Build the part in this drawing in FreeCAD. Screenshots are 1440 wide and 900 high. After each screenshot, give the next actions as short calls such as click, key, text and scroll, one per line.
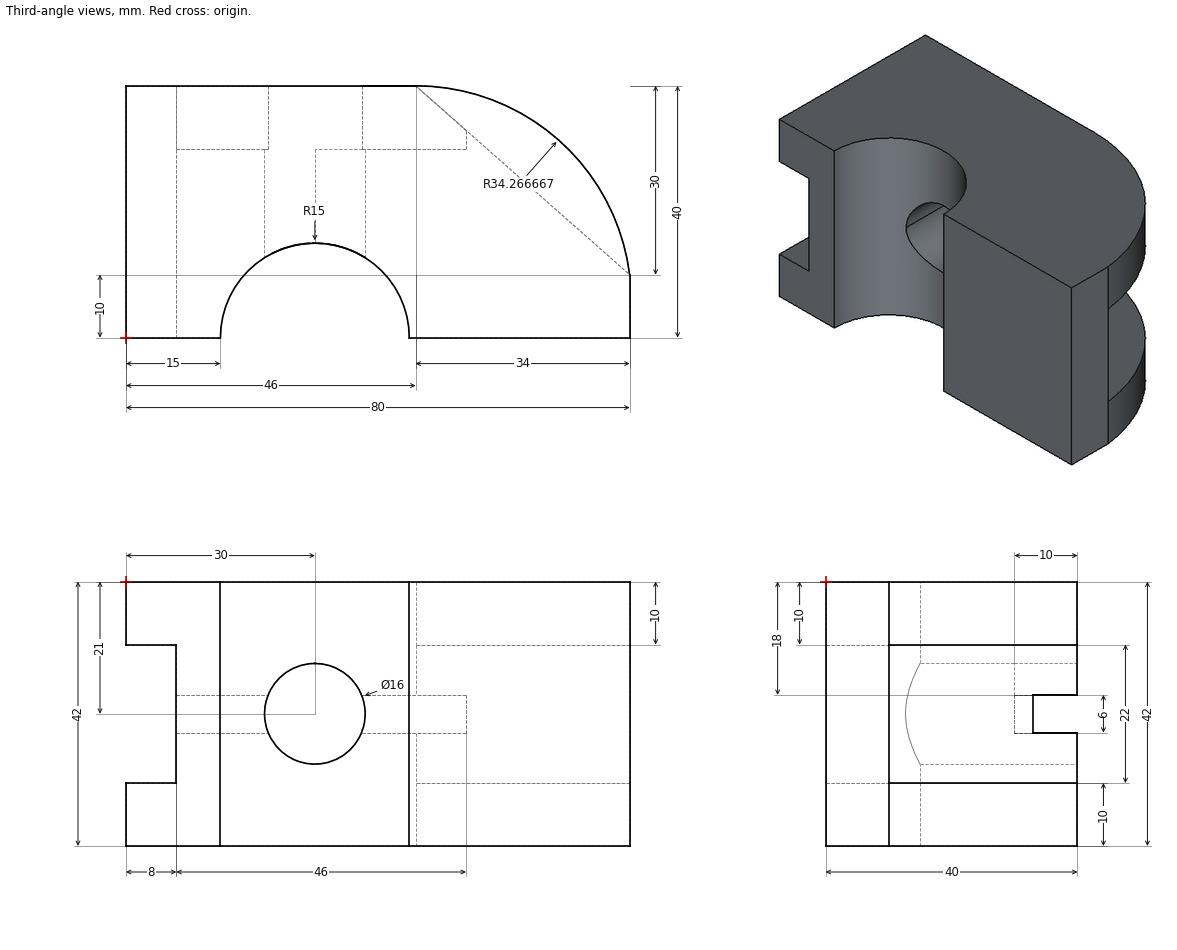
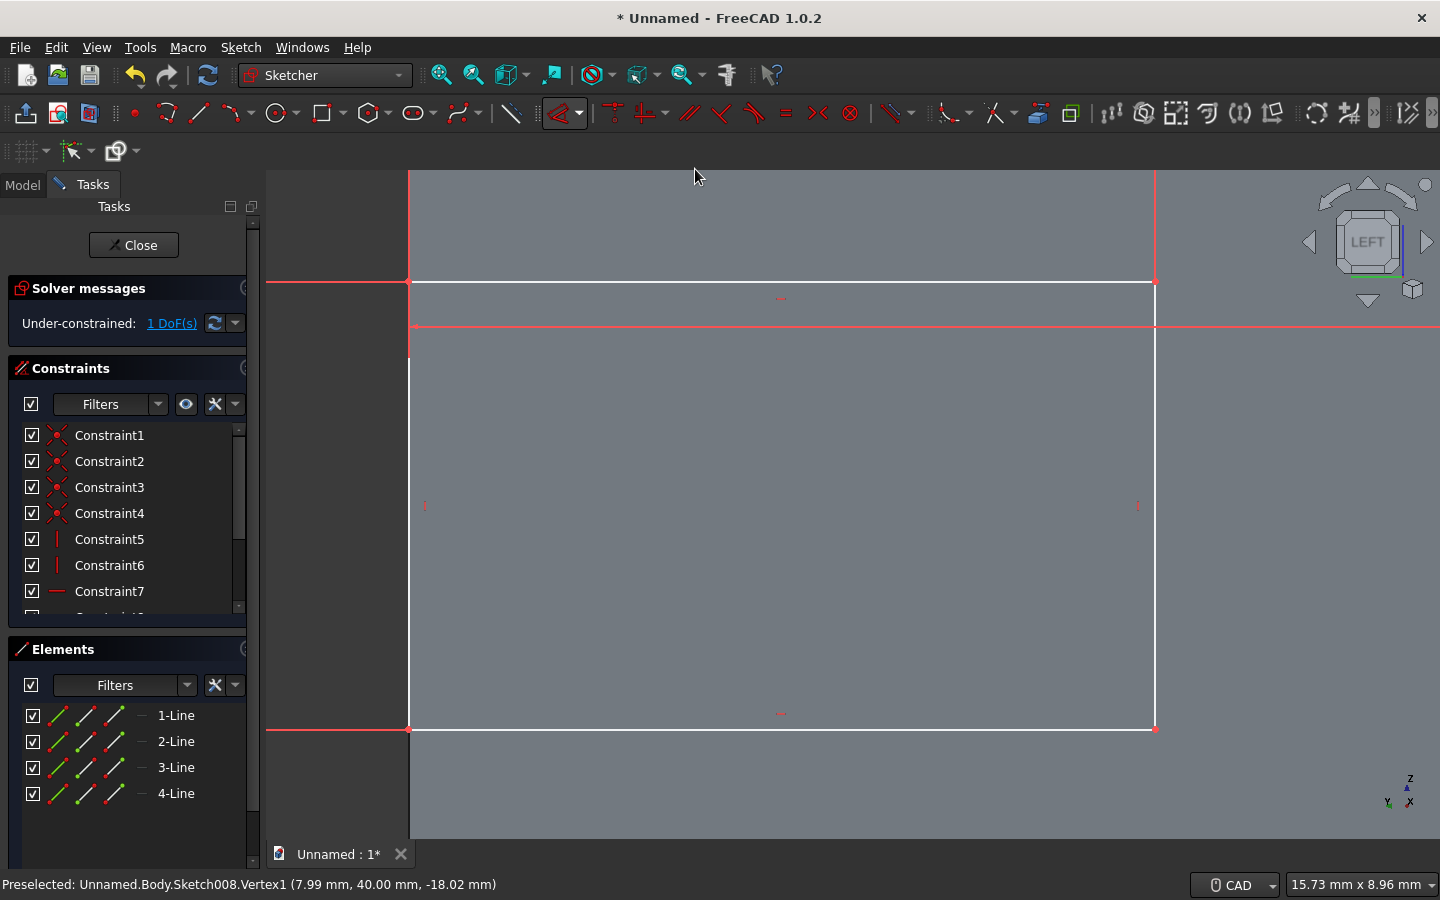
click(409, 282)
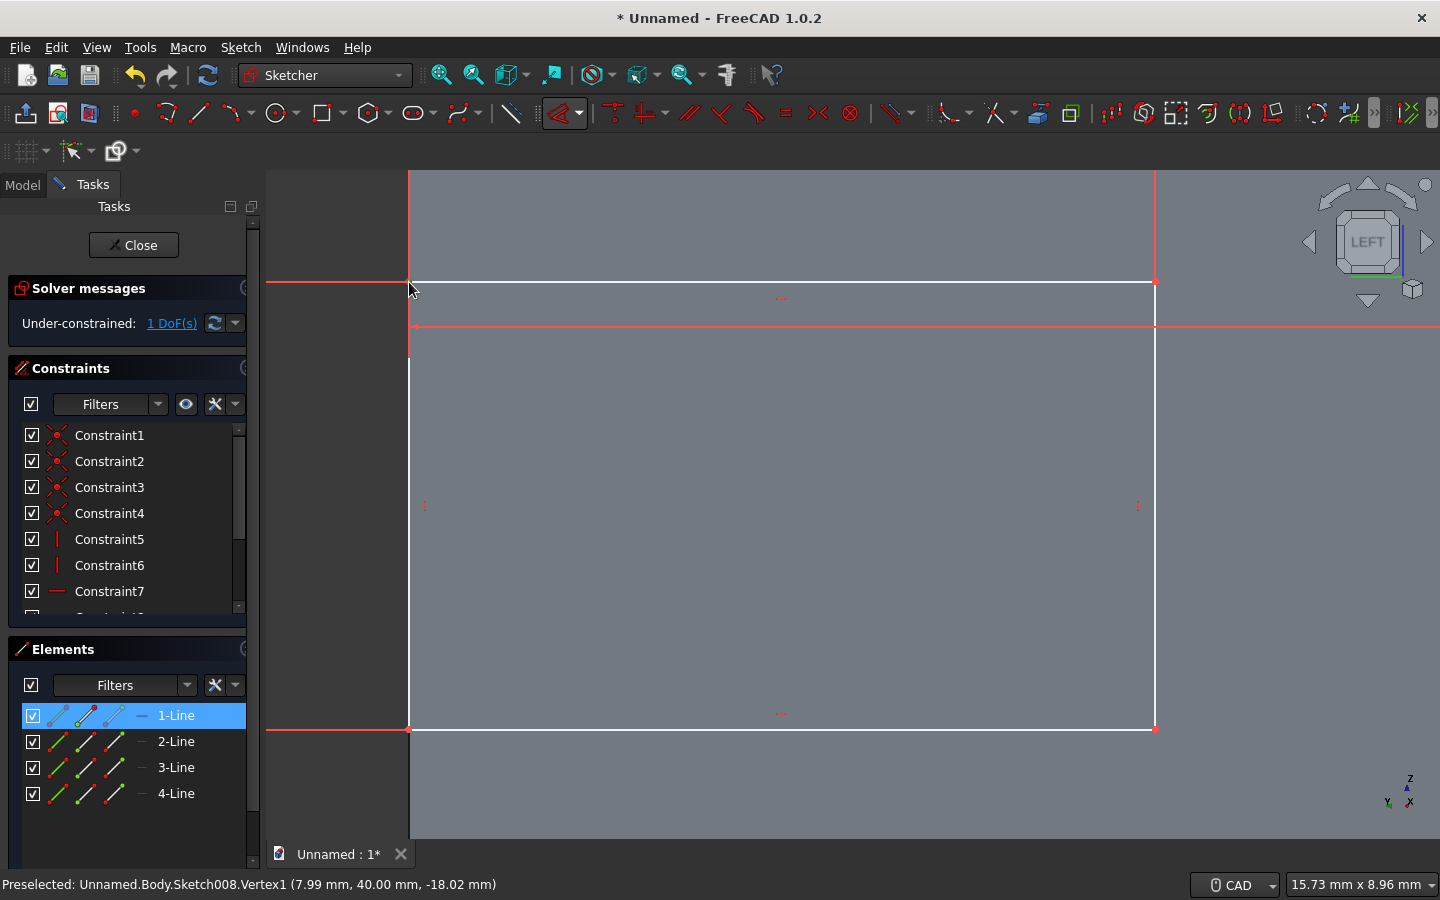
click(582, 114)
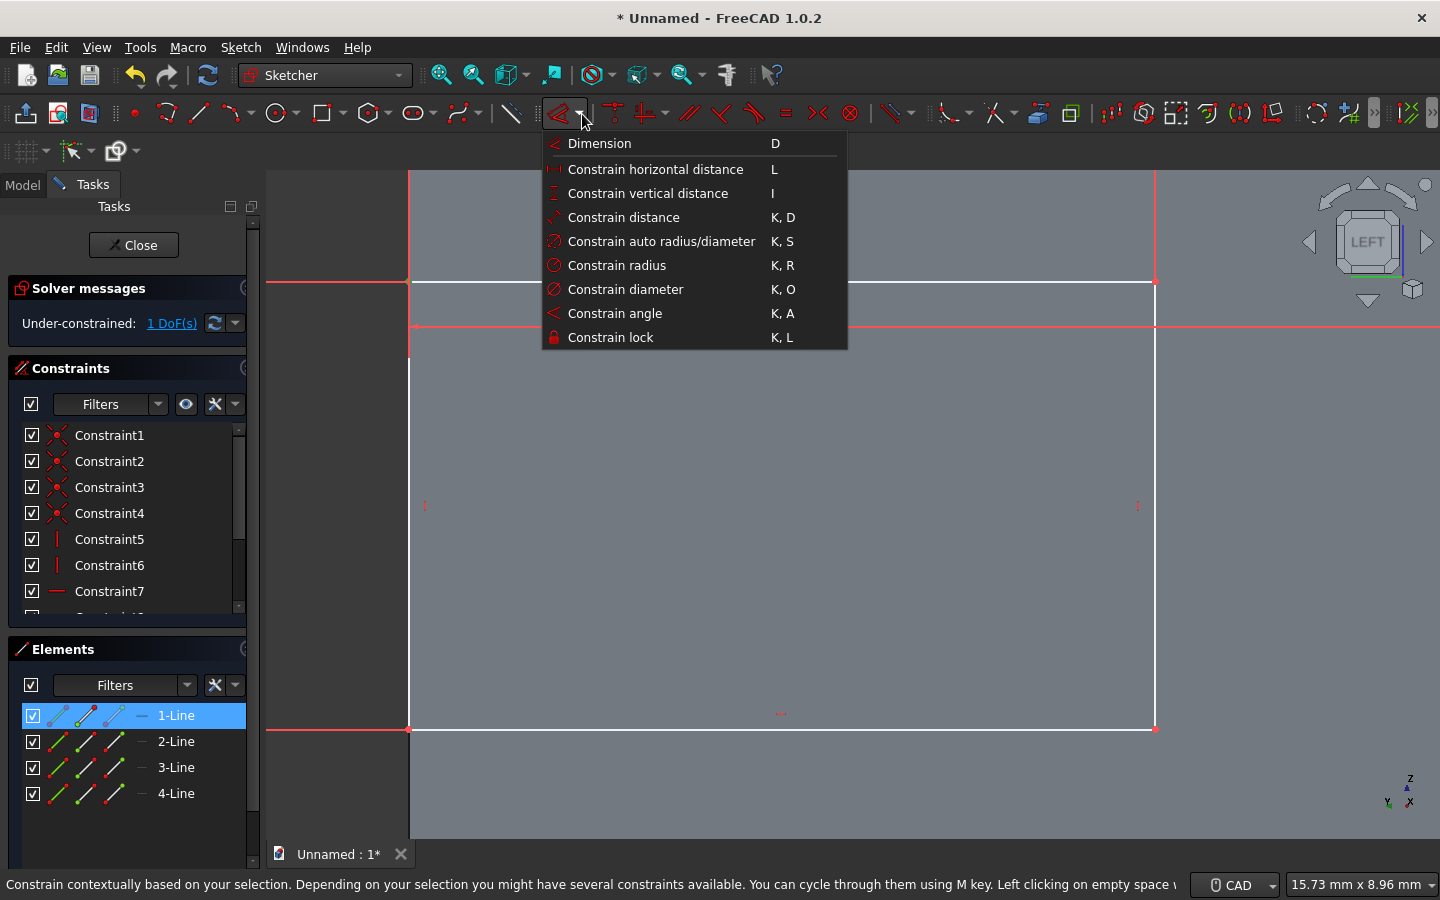
click(695, 193)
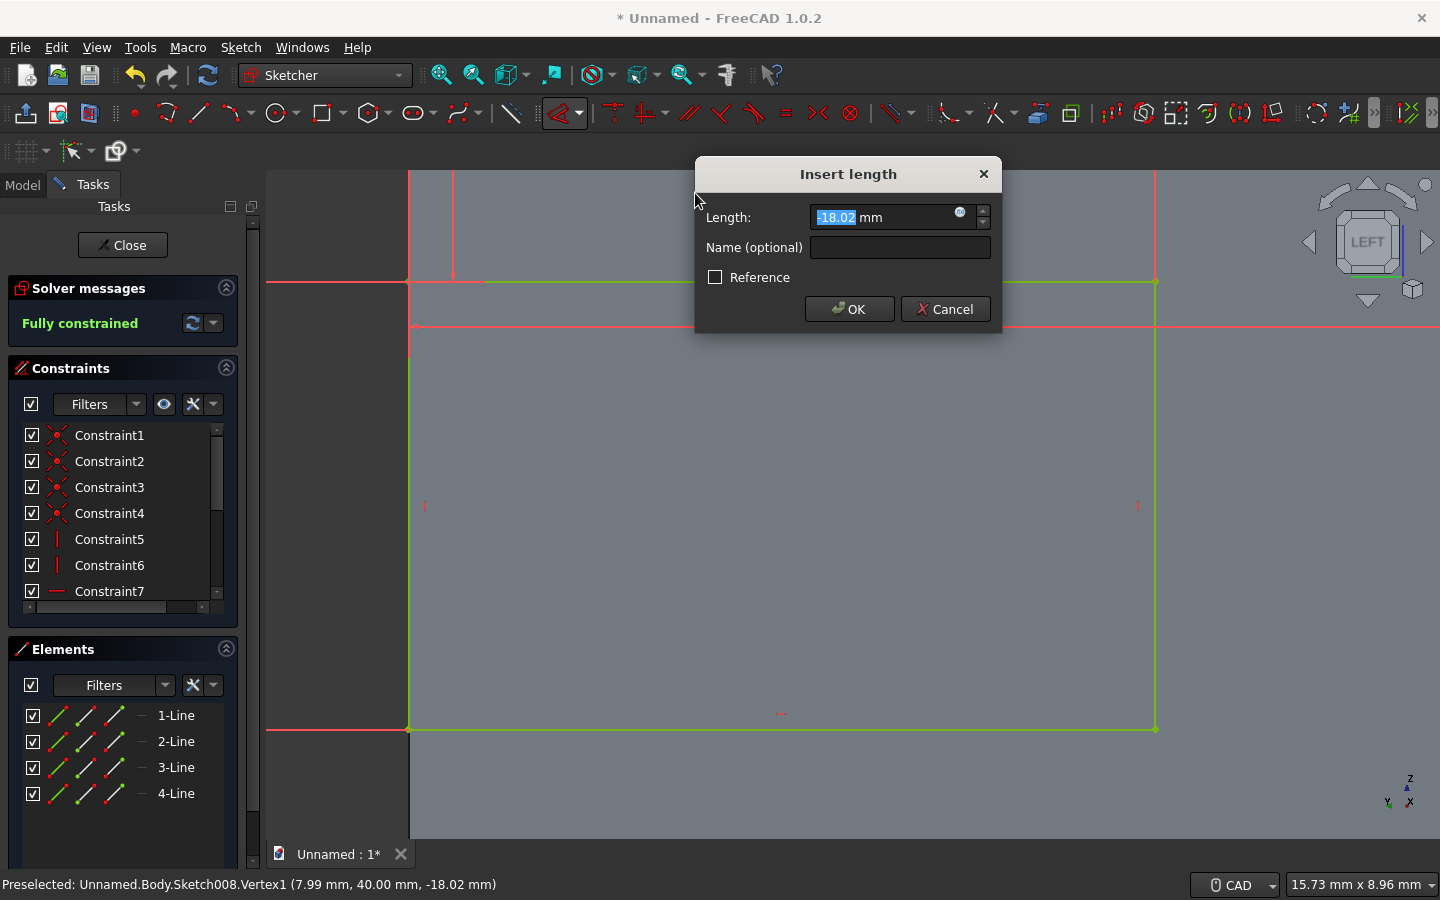
text(-18)
key(Return)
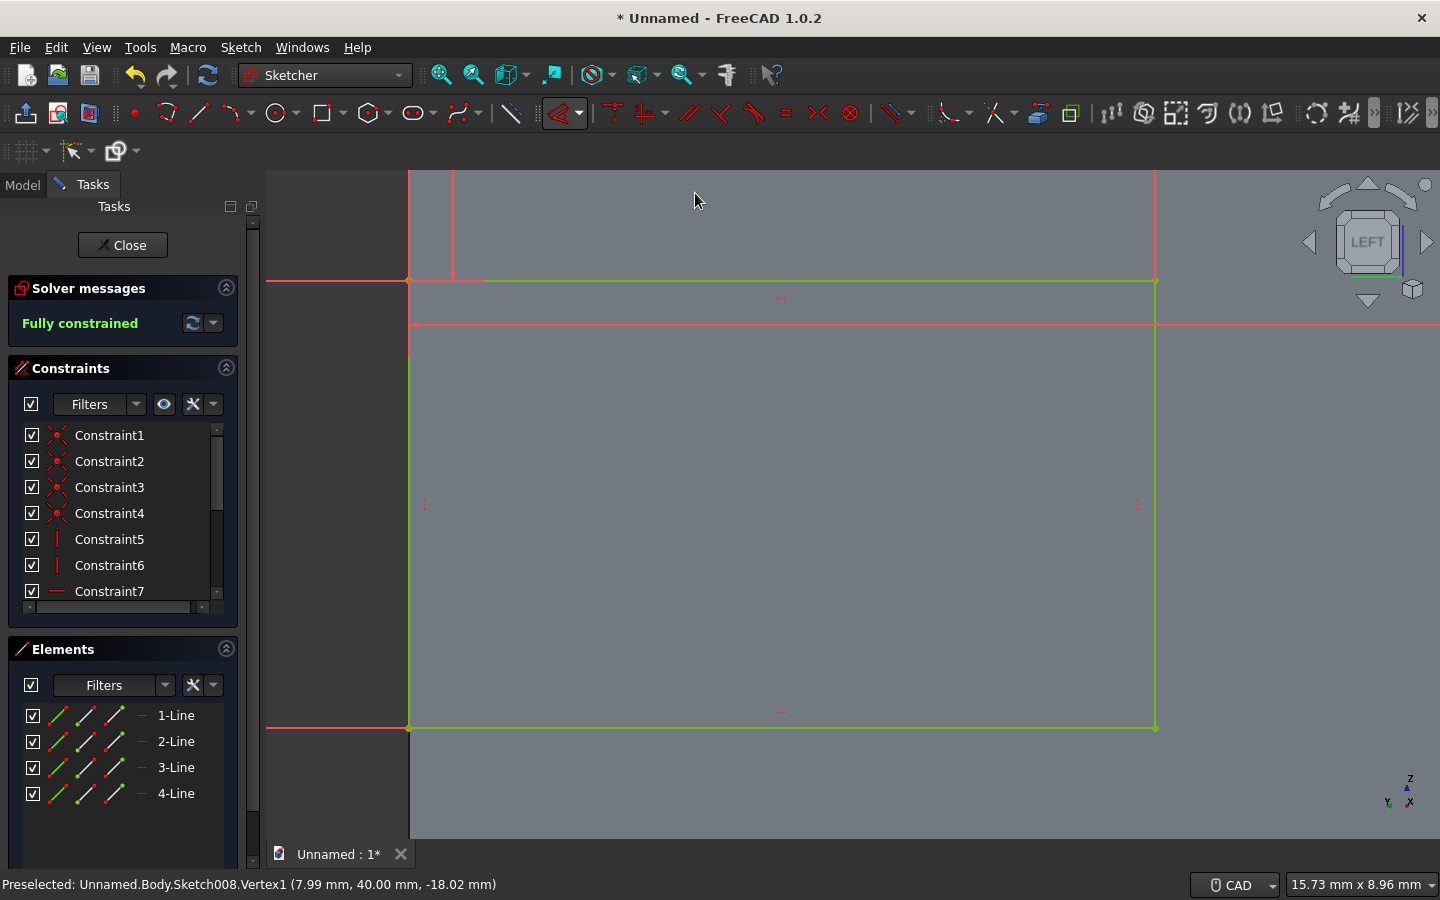
click(123, 245)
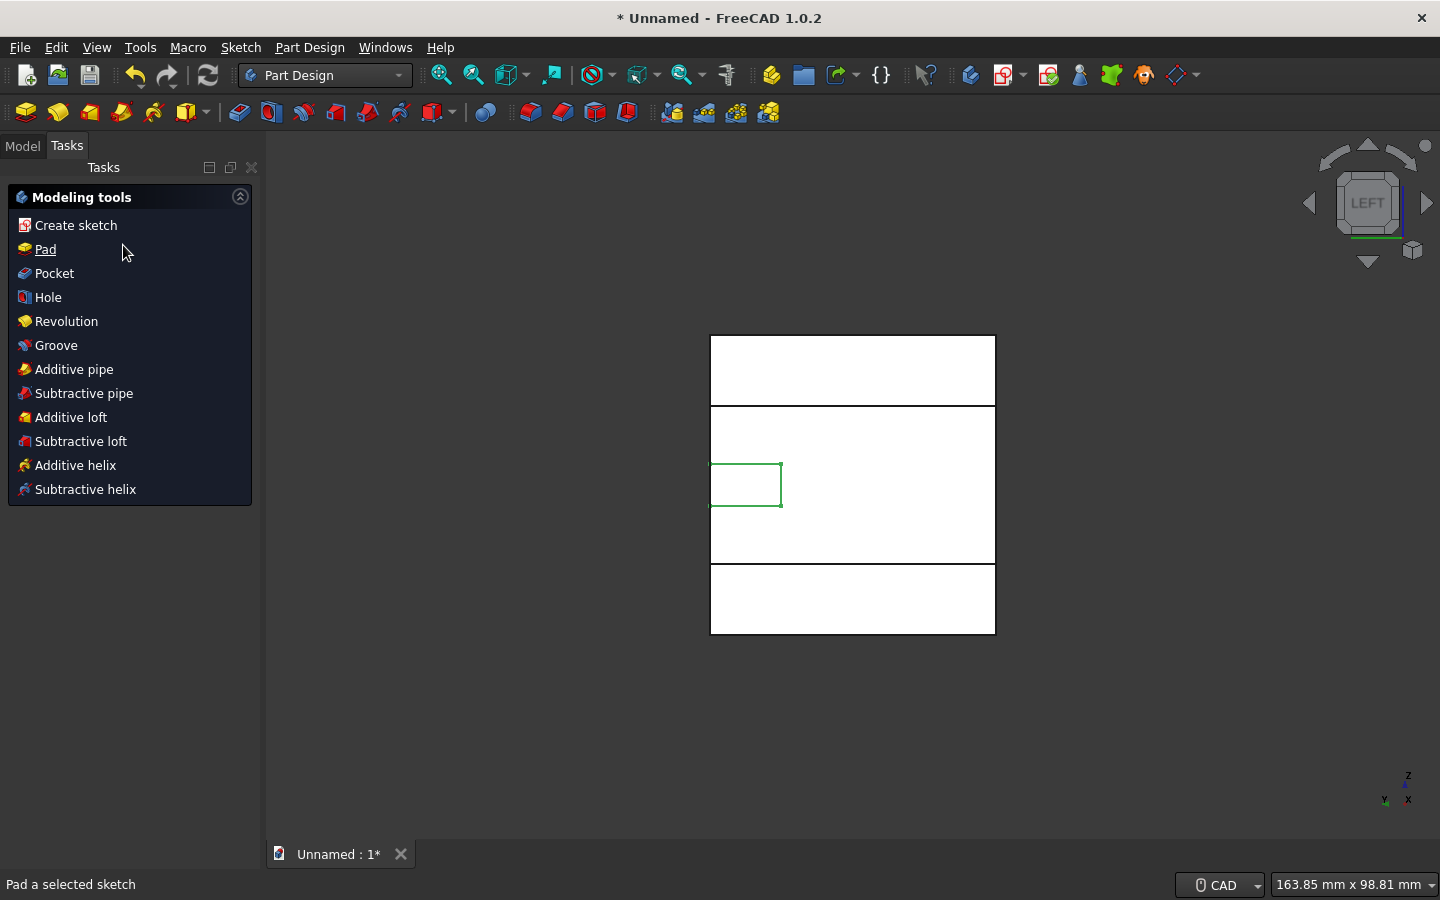
click(240, 112)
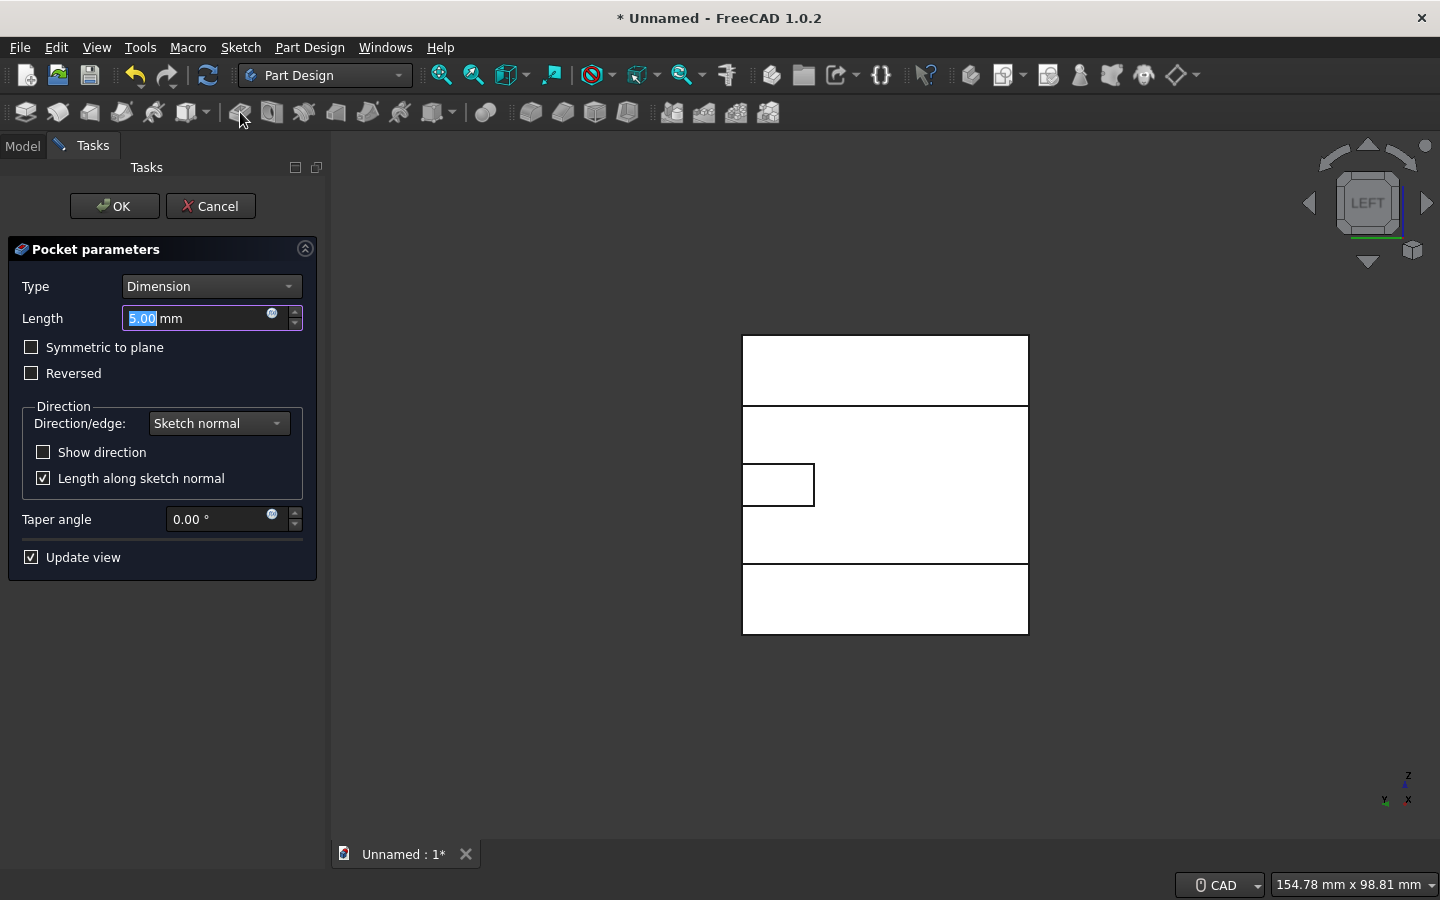
text(46)
key(Tab)